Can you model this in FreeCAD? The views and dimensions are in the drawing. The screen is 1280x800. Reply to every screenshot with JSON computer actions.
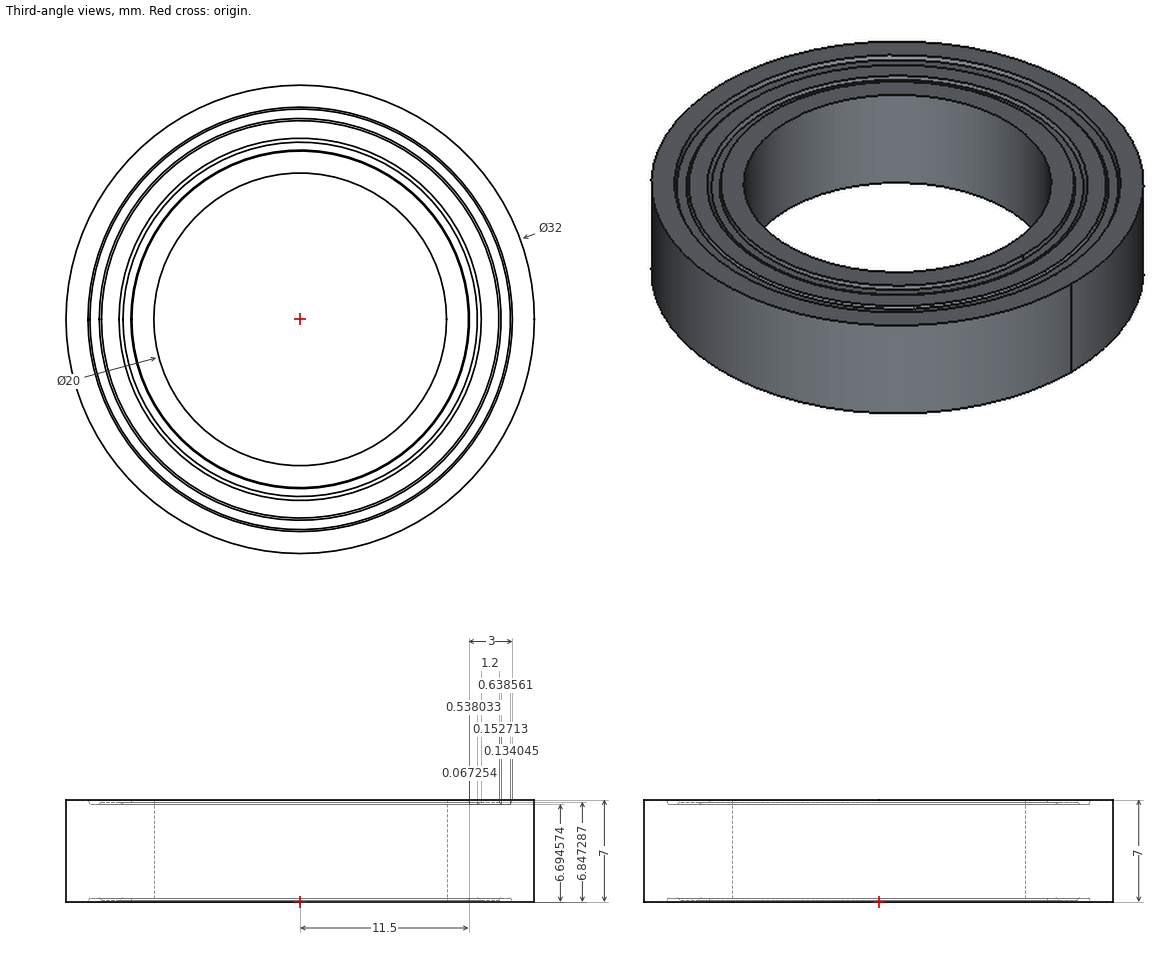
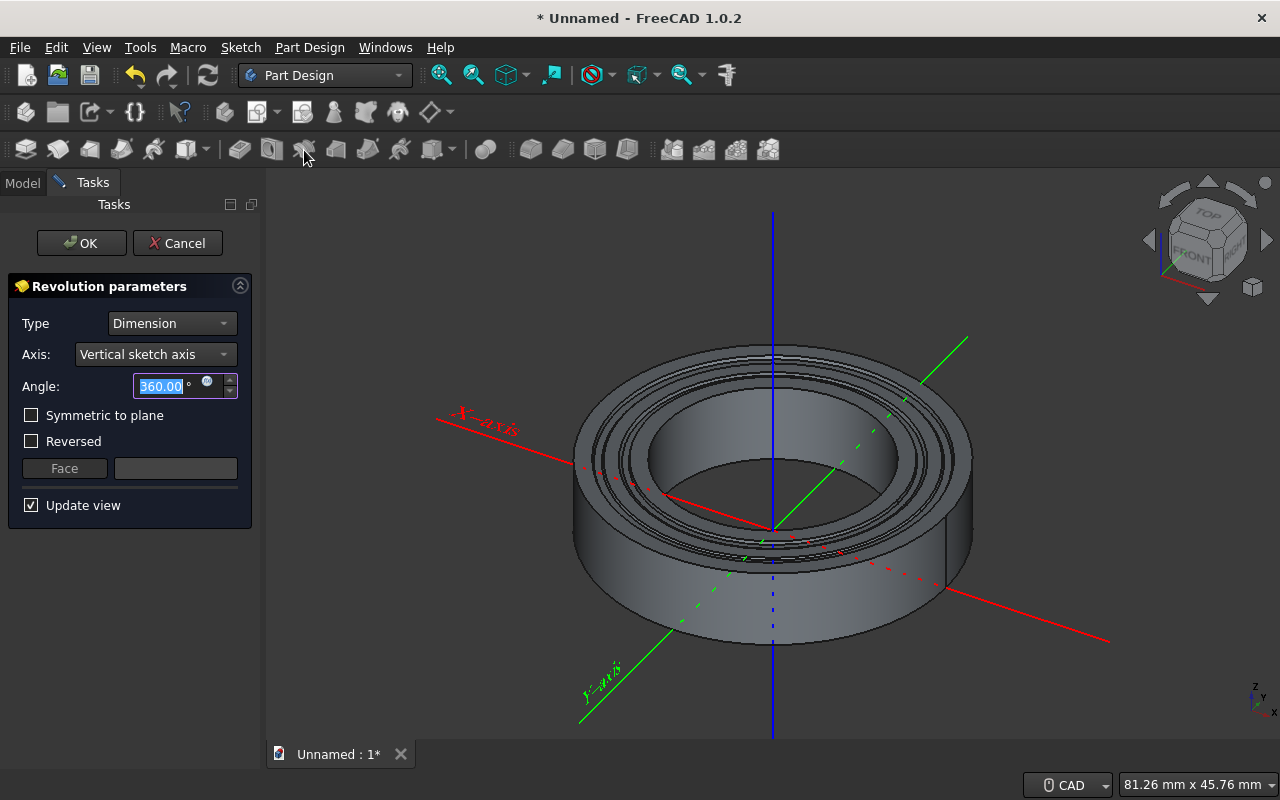
{"action": "left_click", "coordinate": [82, 243]}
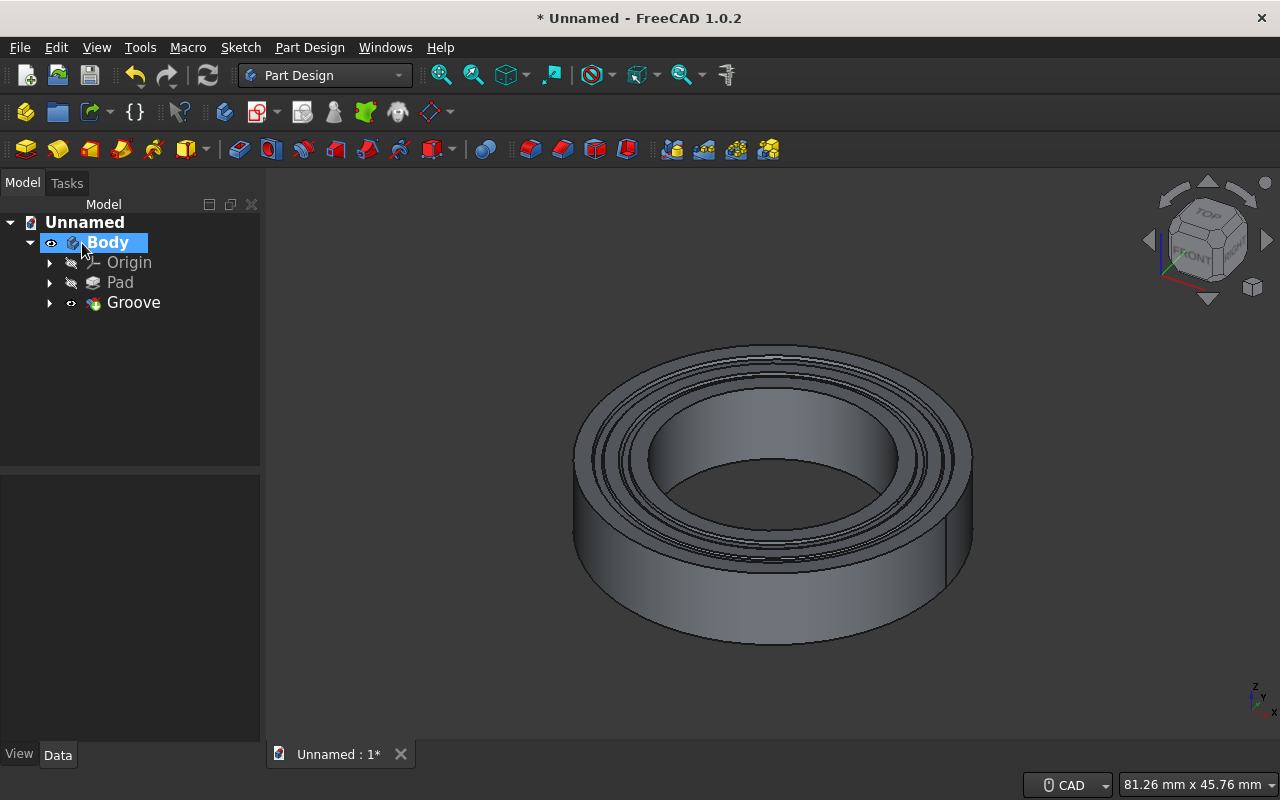
{"action": "left_click", "coordinate": [50, 263]}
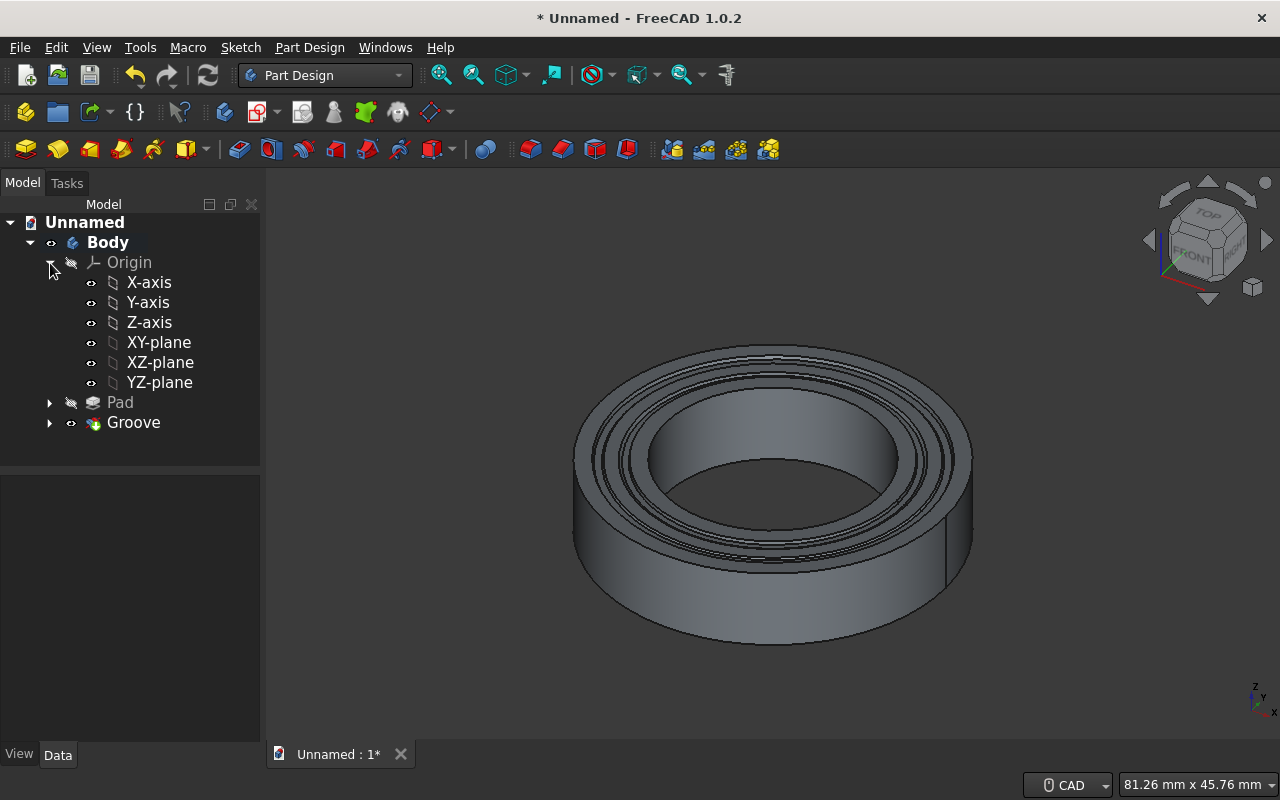
{"action": "left_click", "coordinate": [136, 343]}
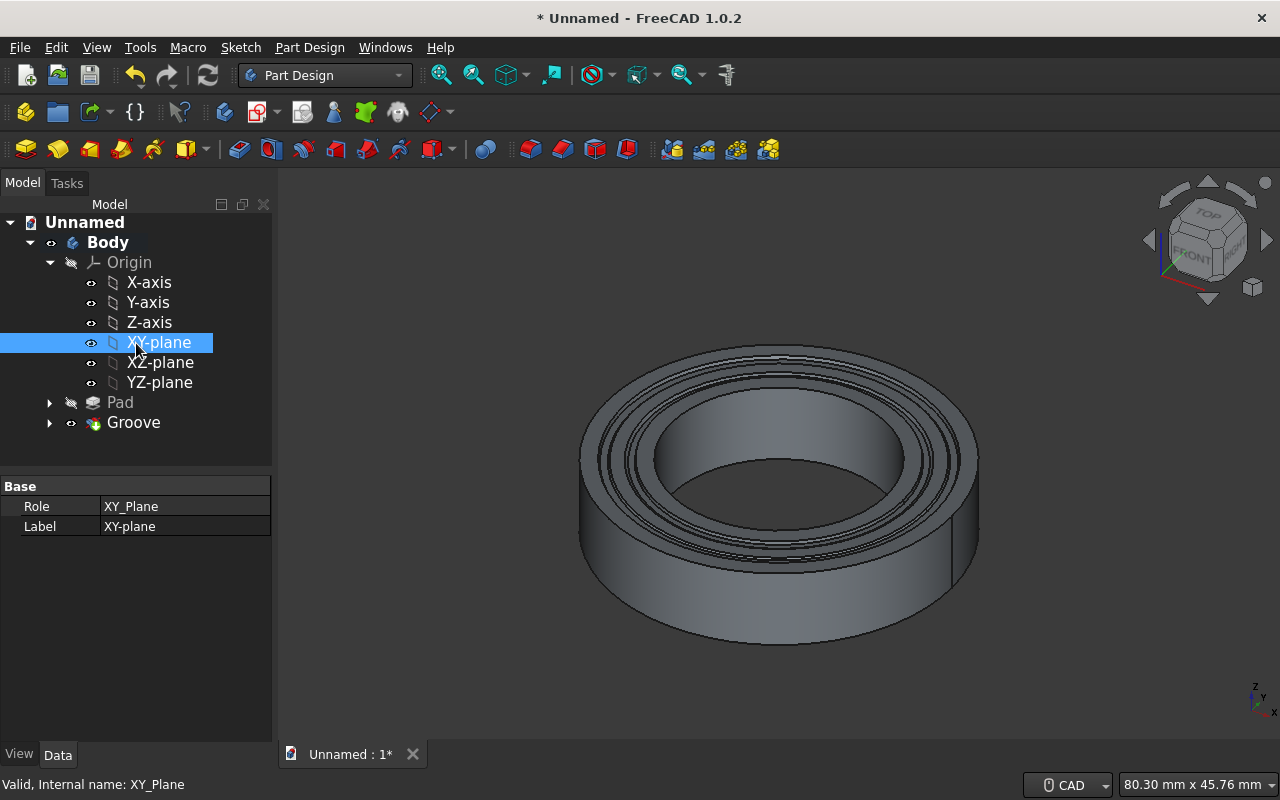
{"action": "left_click", "coordinate": [430, 112]}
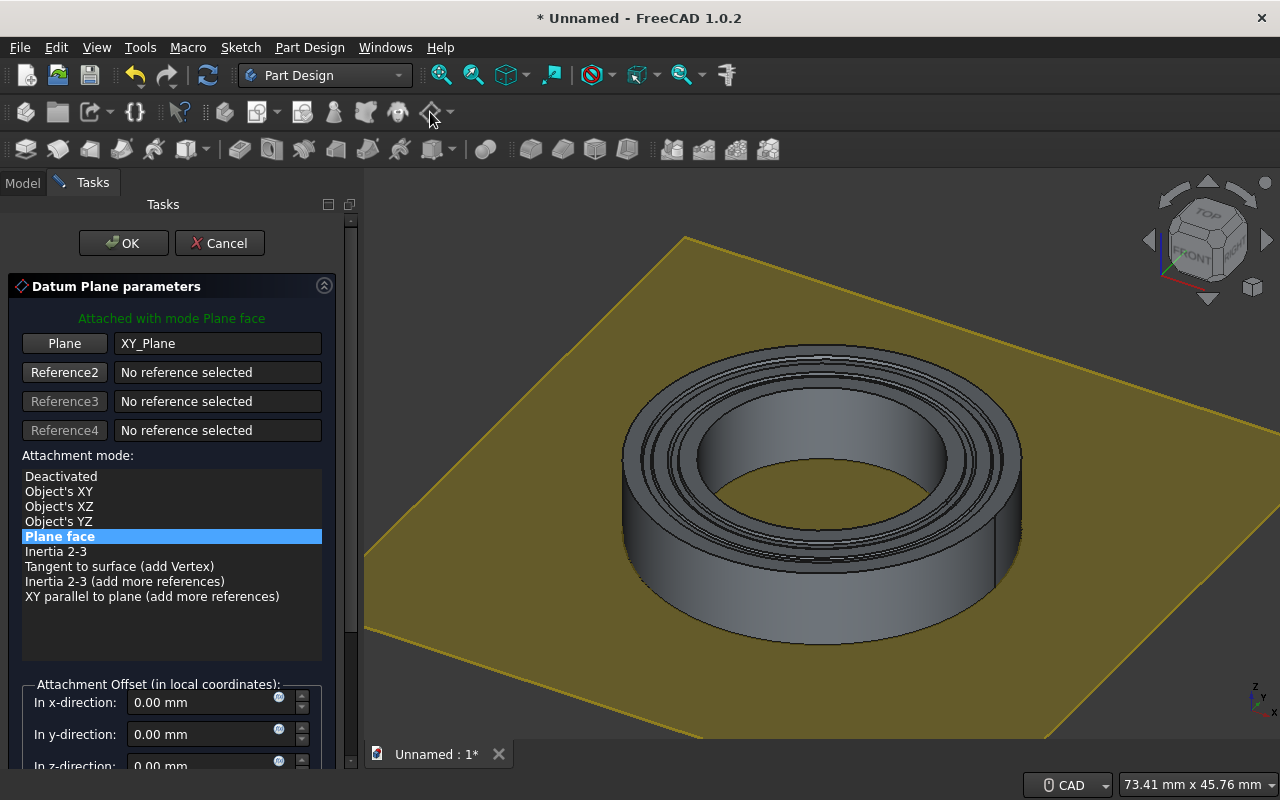
{"action": "scroll", "coordinate": [351, 491], "scroll_direction": "down", "scroll_amount": 2}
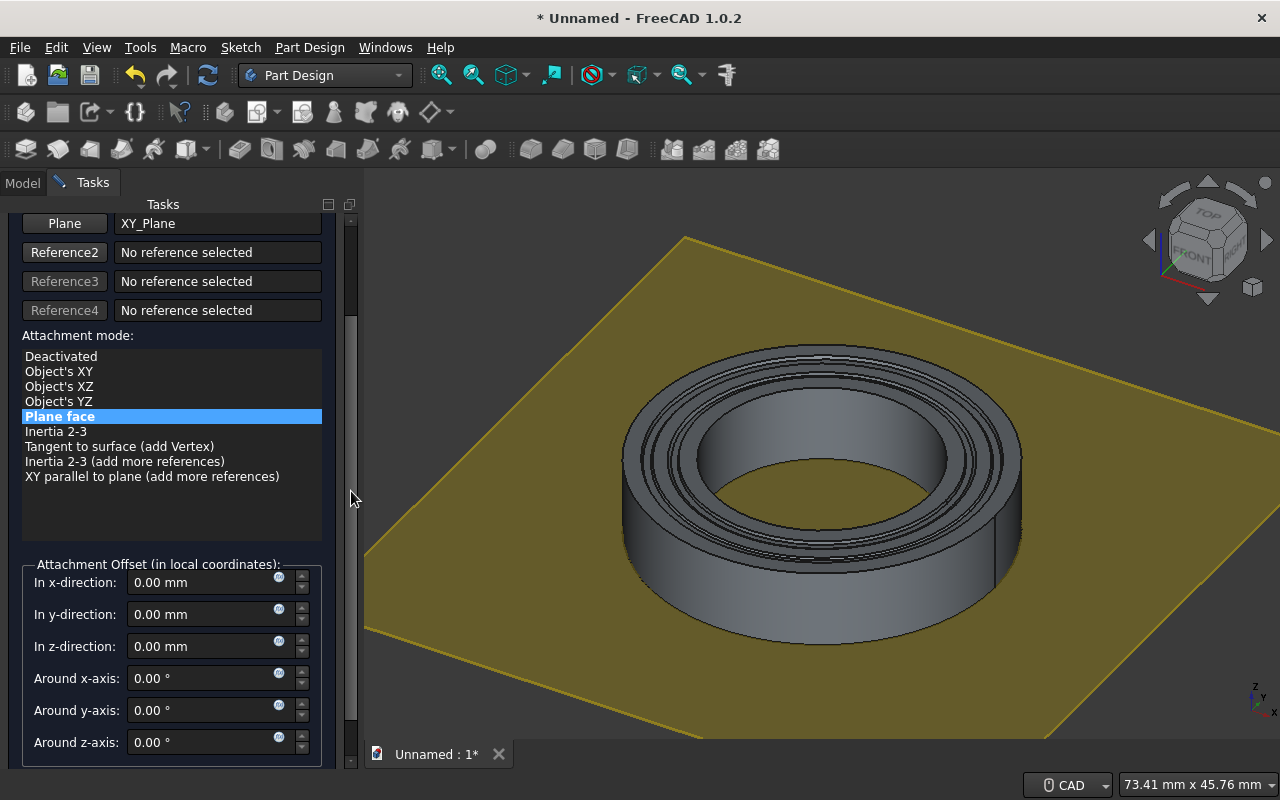
{"action": "triple_click", "coordinate": [210, 646]}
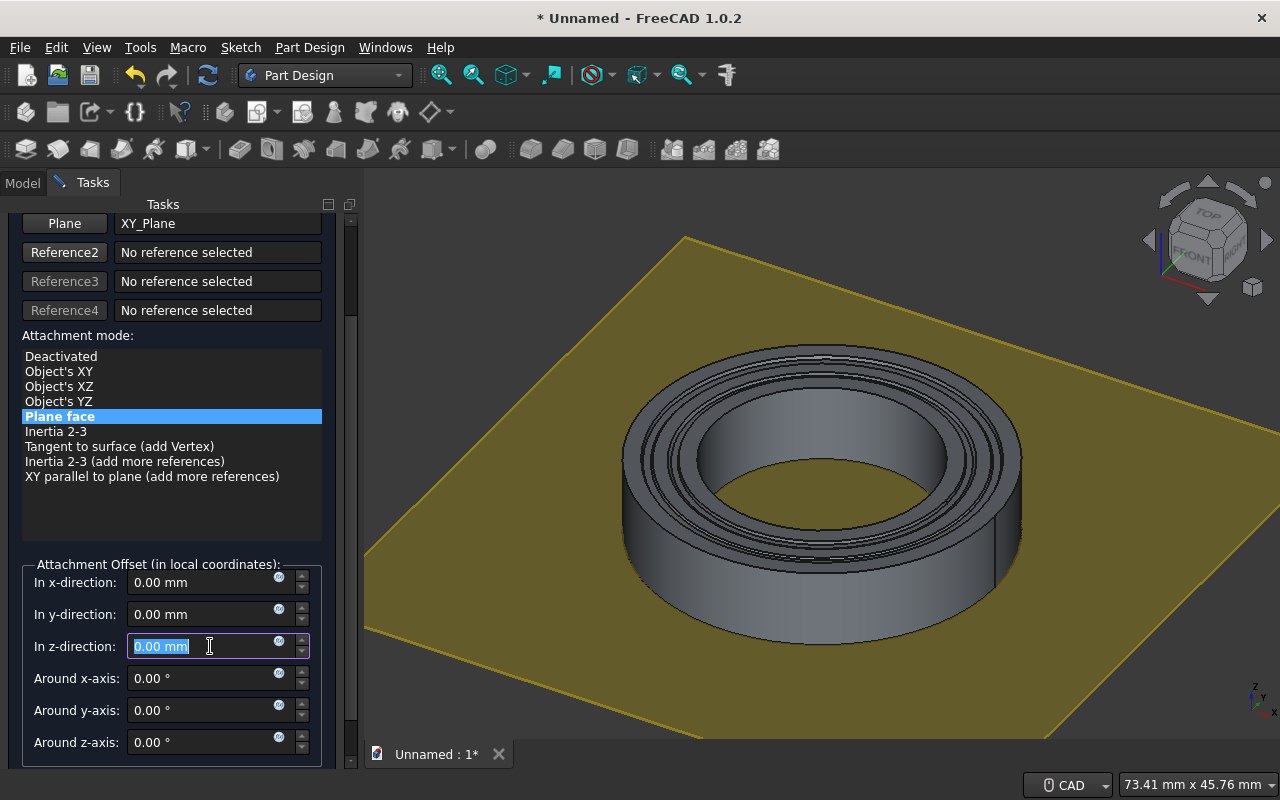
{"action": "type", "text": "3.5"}
{"action": "key", "text": "Tab"}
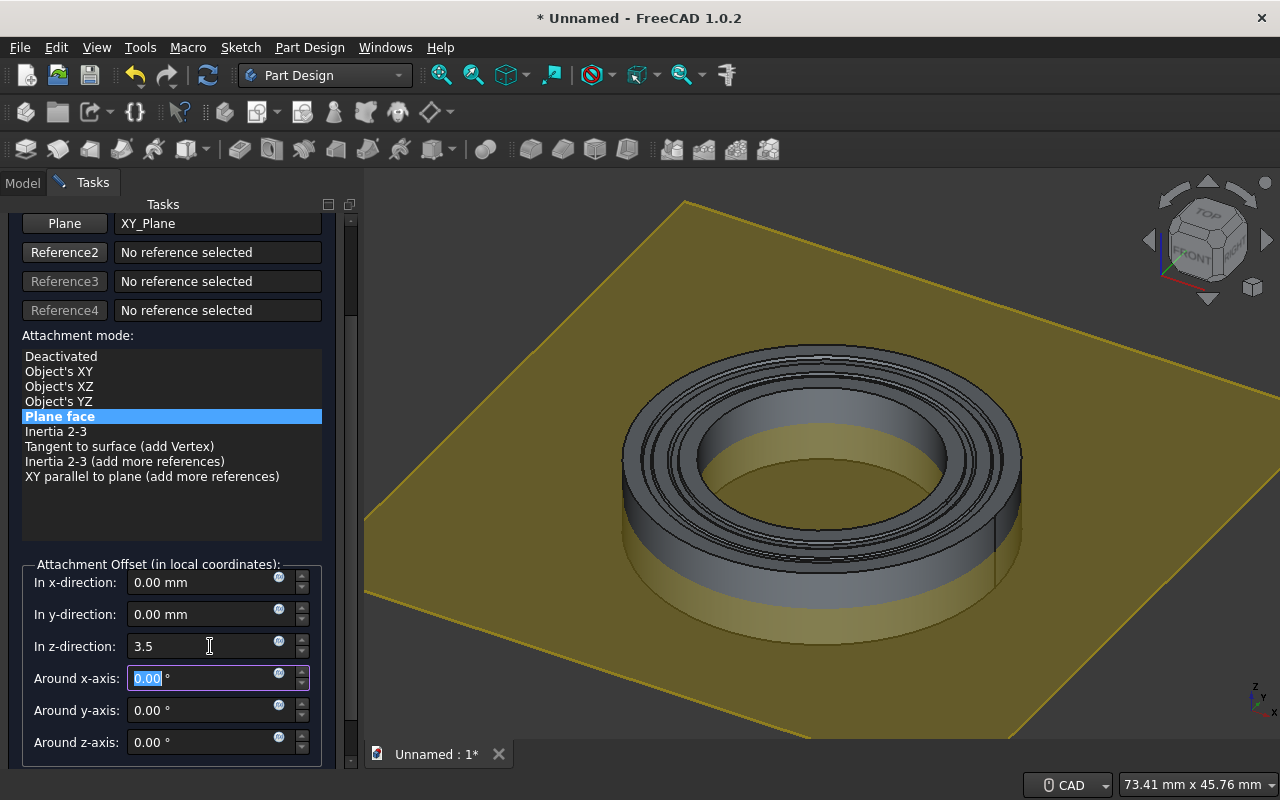
{"action": "scroll", "coordinate": [351, 491], "scroll_direction": "up", "scroll_amount": 3}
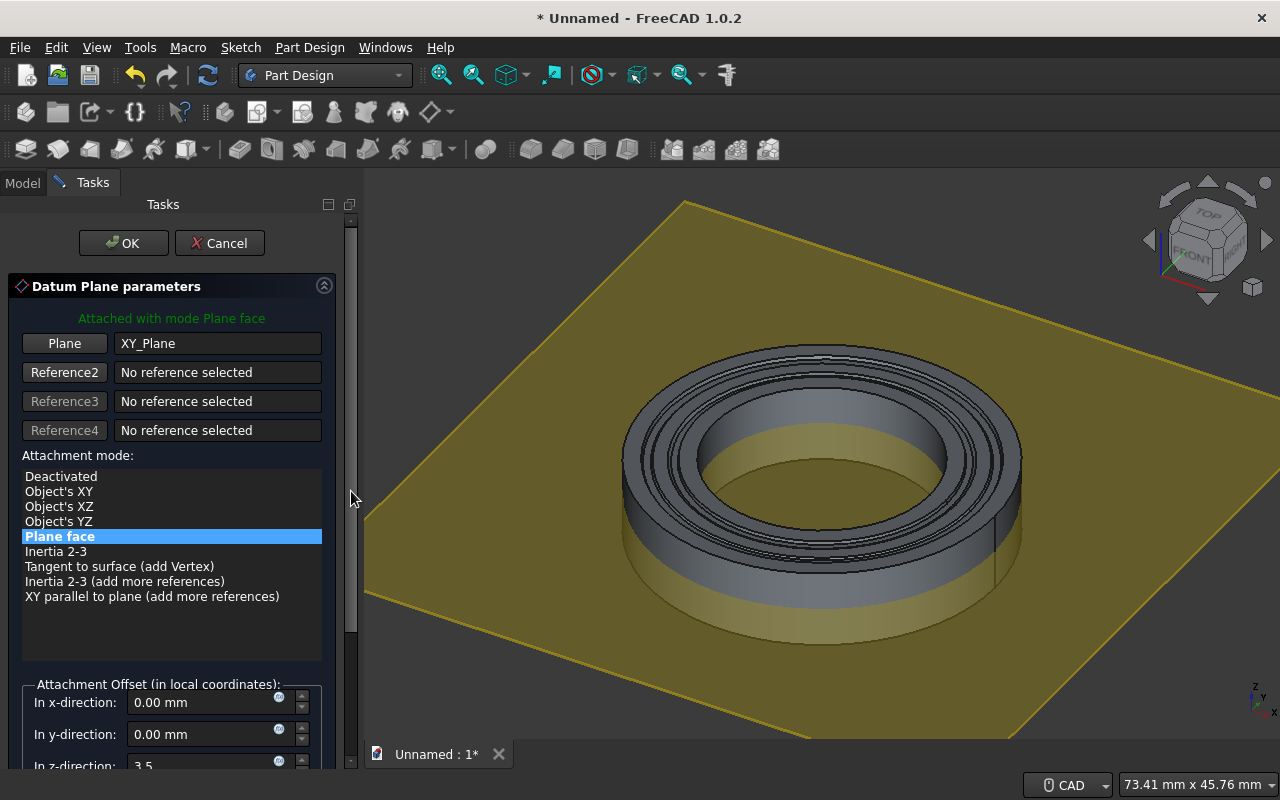
{"action": "left_click", "coordinate": [124, 243]}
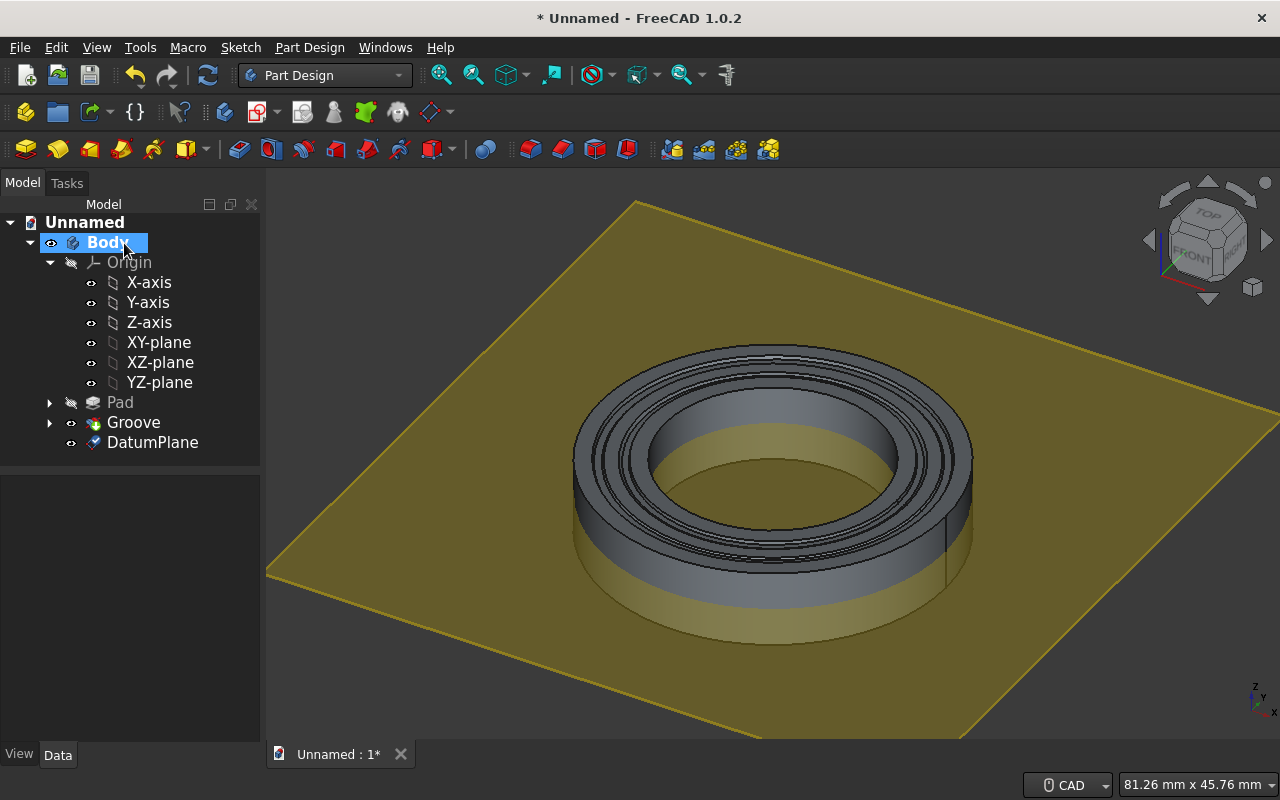
{"action": "left_click", "coordinate": [116, 423]}